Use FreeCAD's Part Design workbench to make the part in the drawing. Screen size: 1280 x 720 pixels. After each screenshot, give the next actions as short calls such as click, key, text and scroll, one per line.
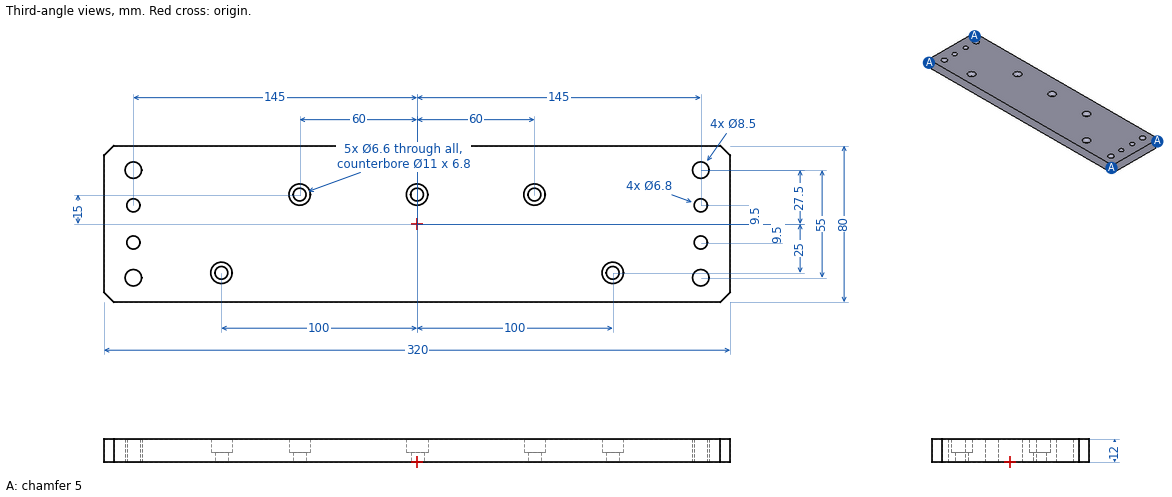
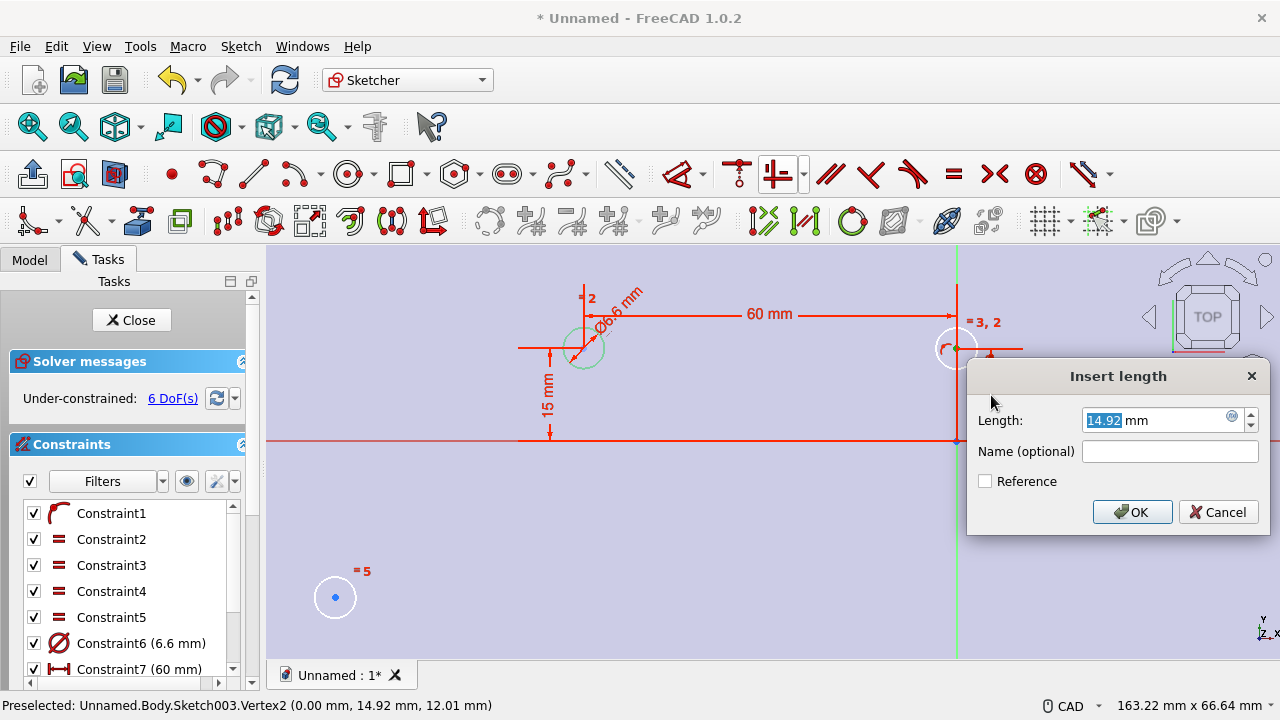
text(15)
key(Return)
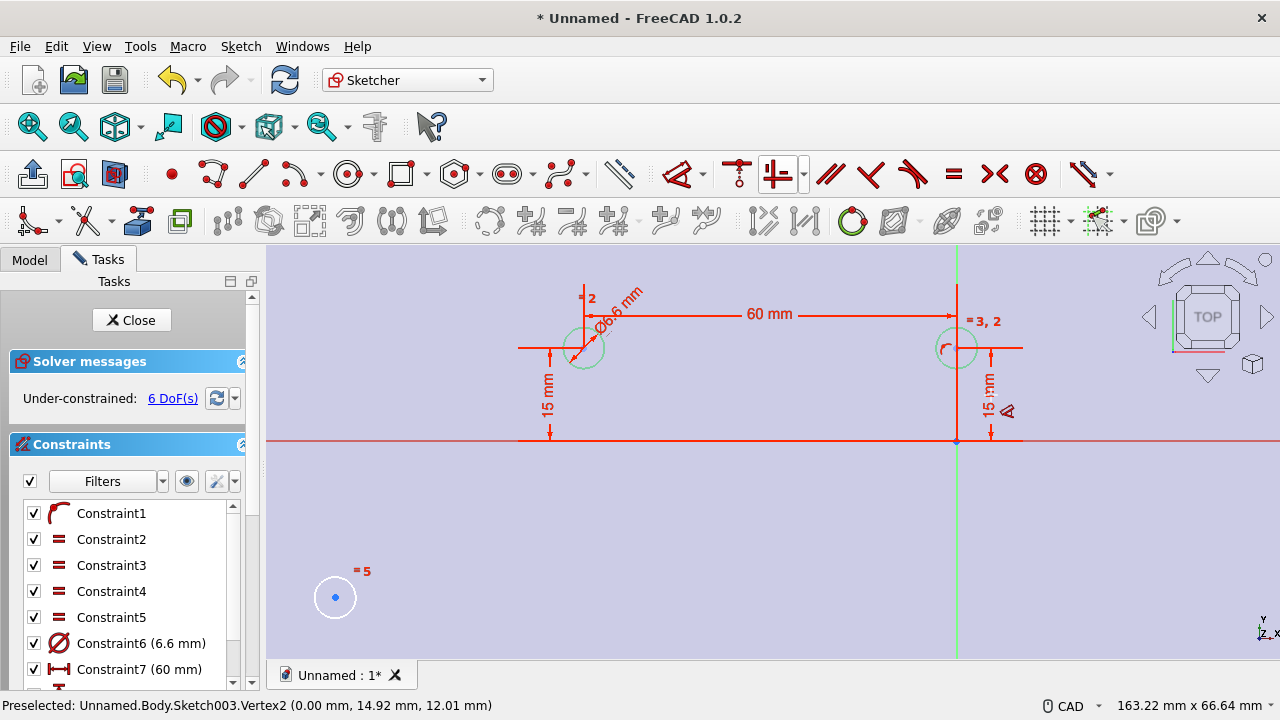
scroll(499, 435, down, 4)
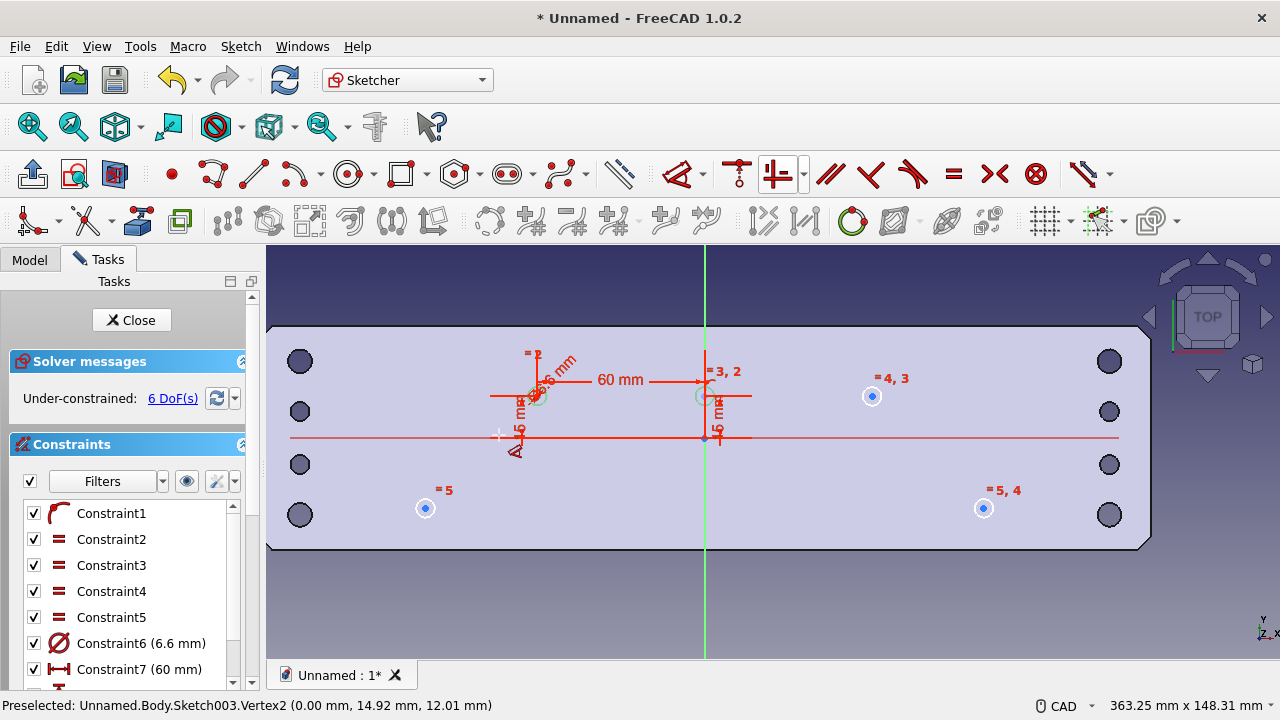
click(872, 396)
click(788, 362)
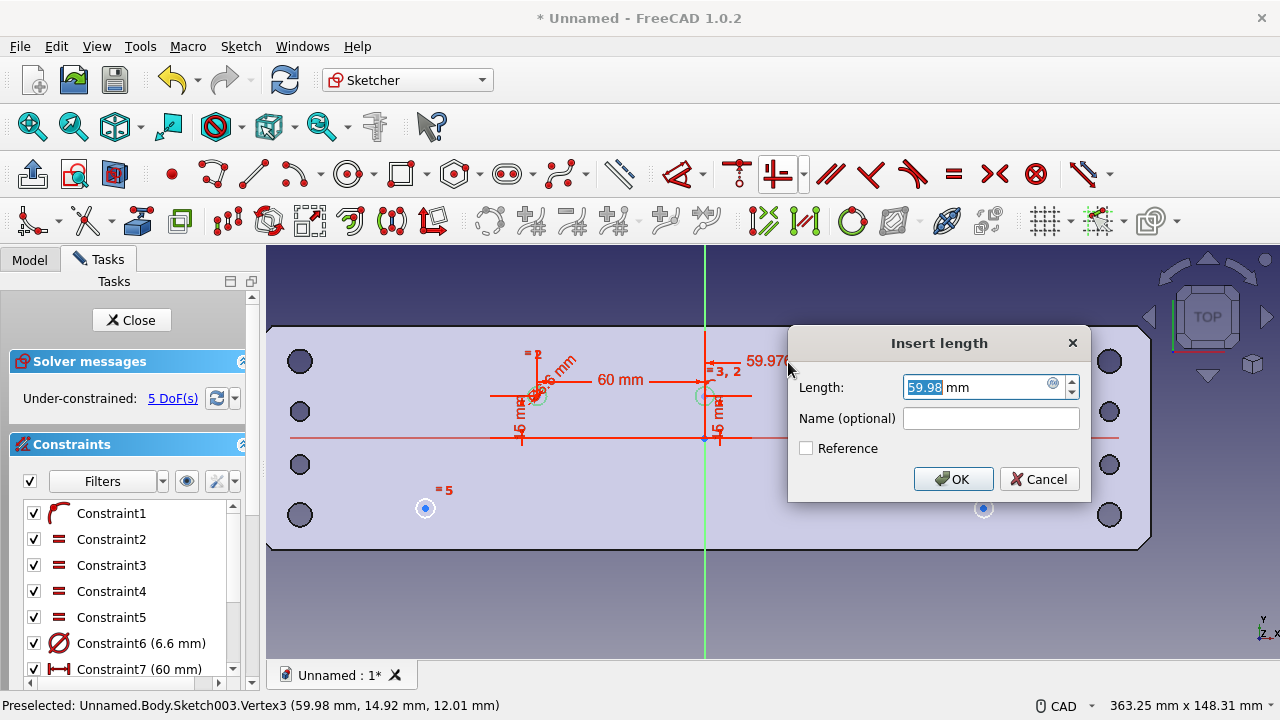
text(60)
key(Return)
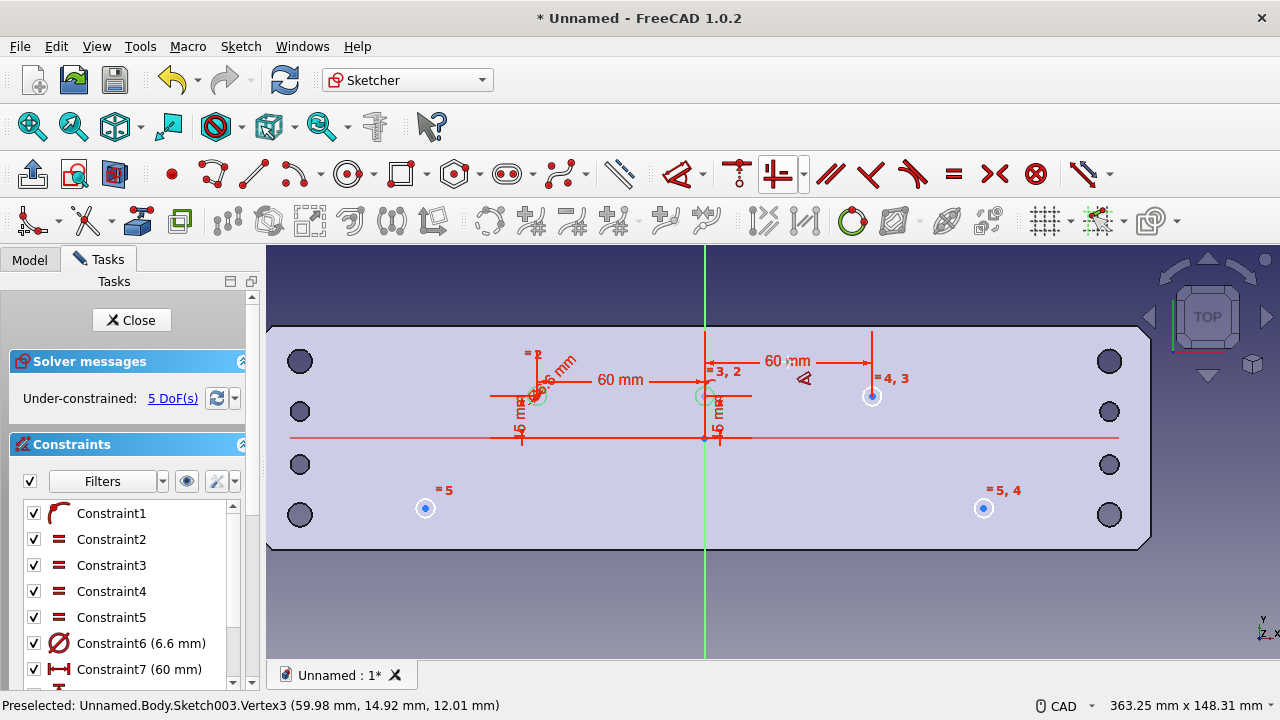
click(872, 396)
click(906, 417)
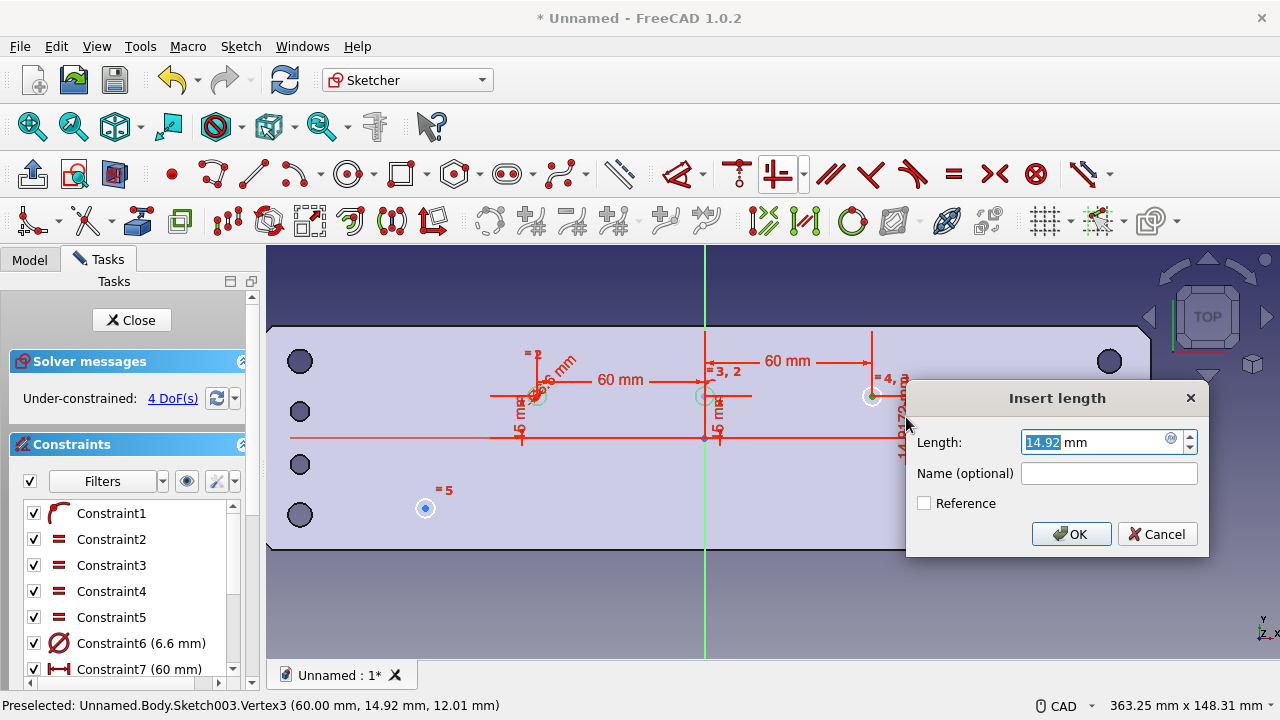
text(15)
key(Return)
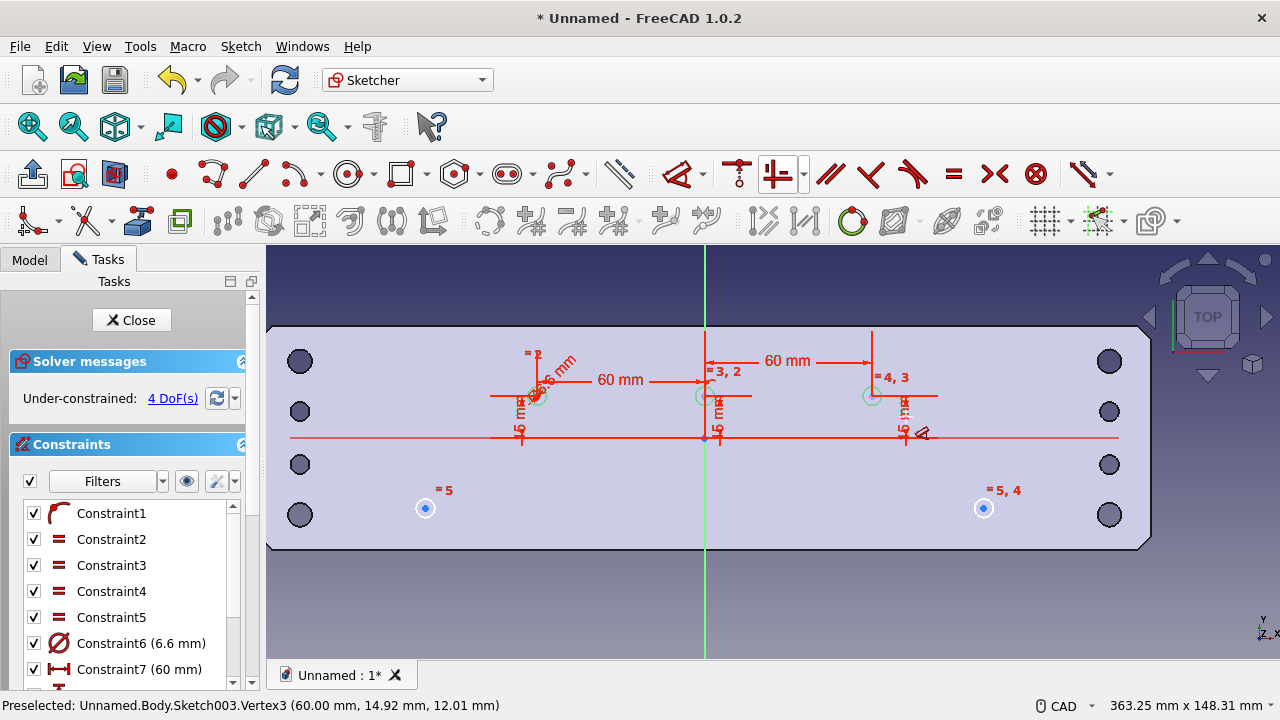
click(984, 508)
click(1018, 473)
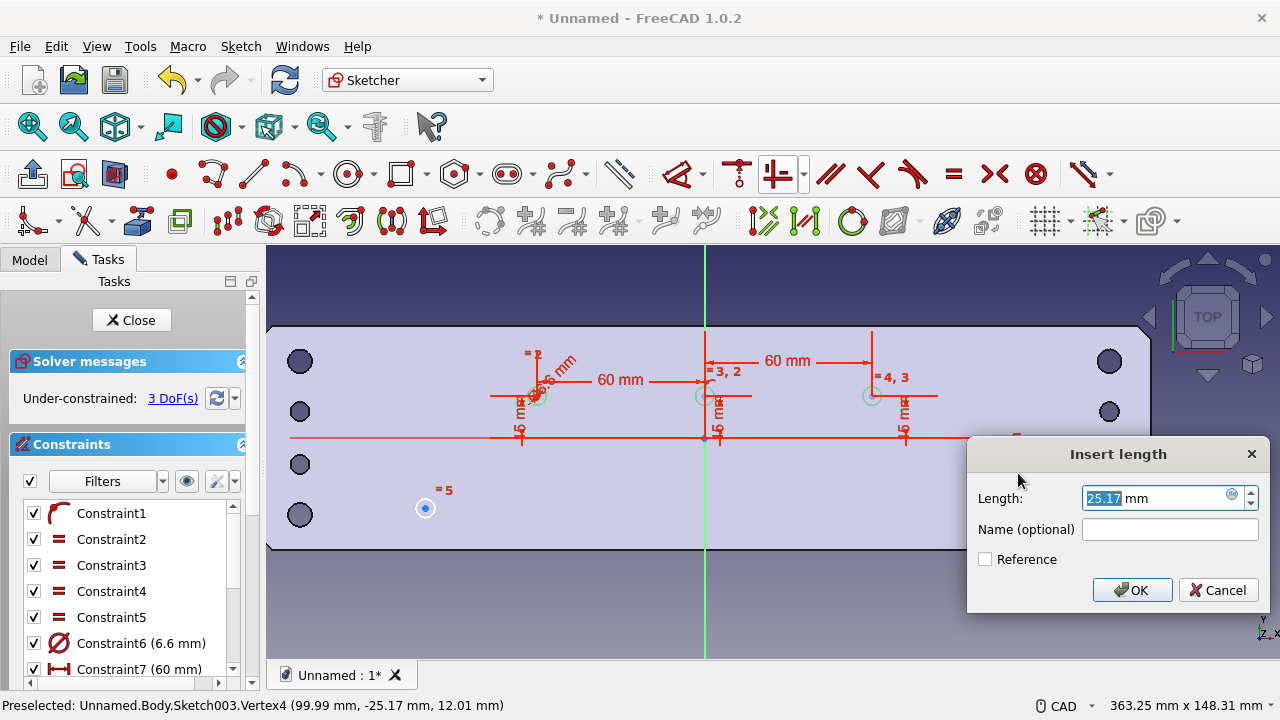
text(25)
key(Return)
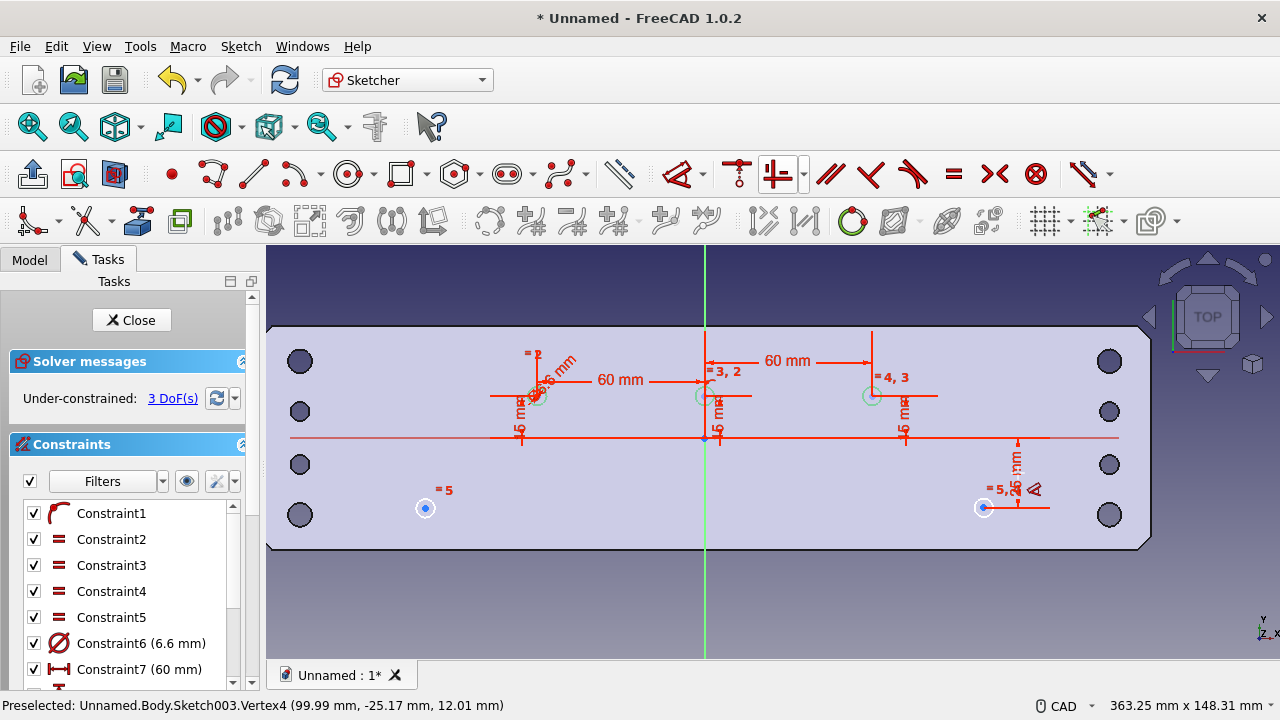
click(426, 508)
click(392, 473)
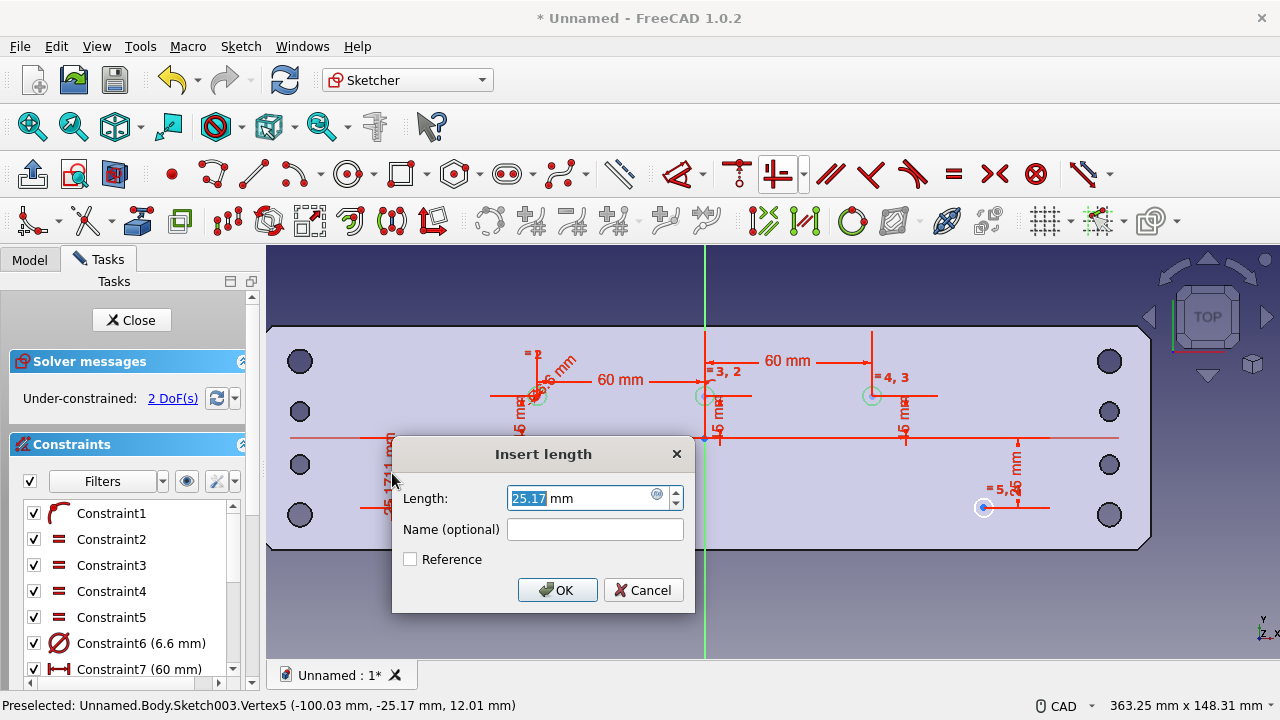
text(25)
key(Return)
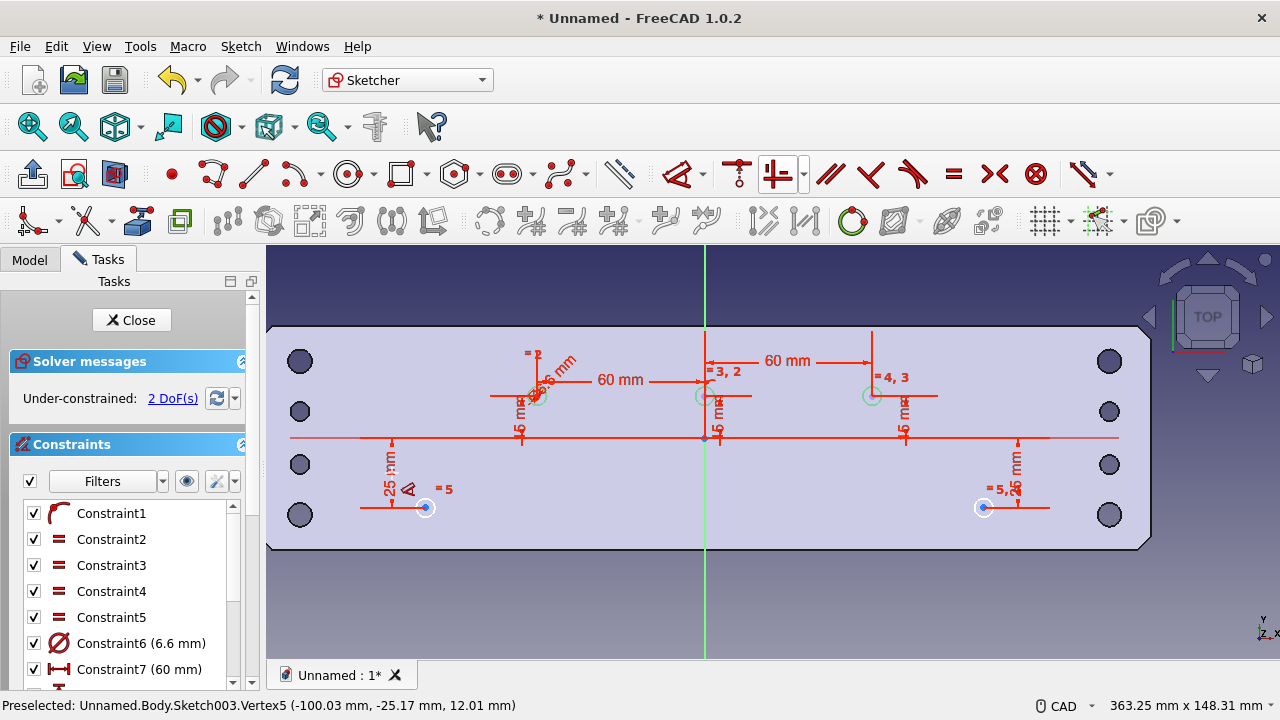
click(984, 508)
click(844, 542)